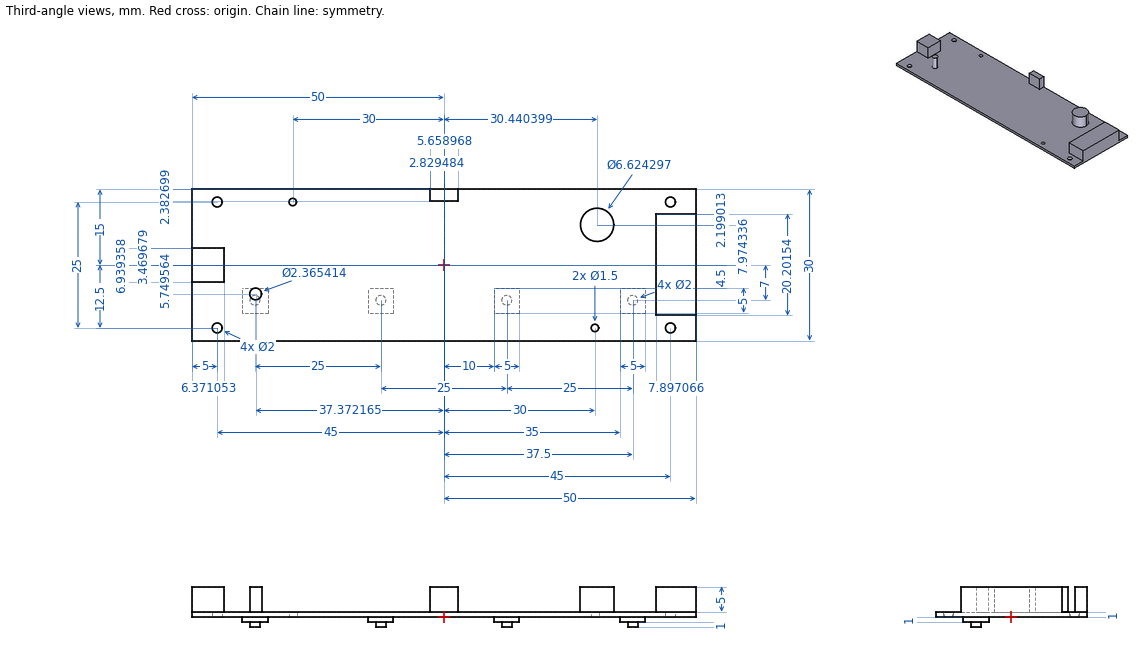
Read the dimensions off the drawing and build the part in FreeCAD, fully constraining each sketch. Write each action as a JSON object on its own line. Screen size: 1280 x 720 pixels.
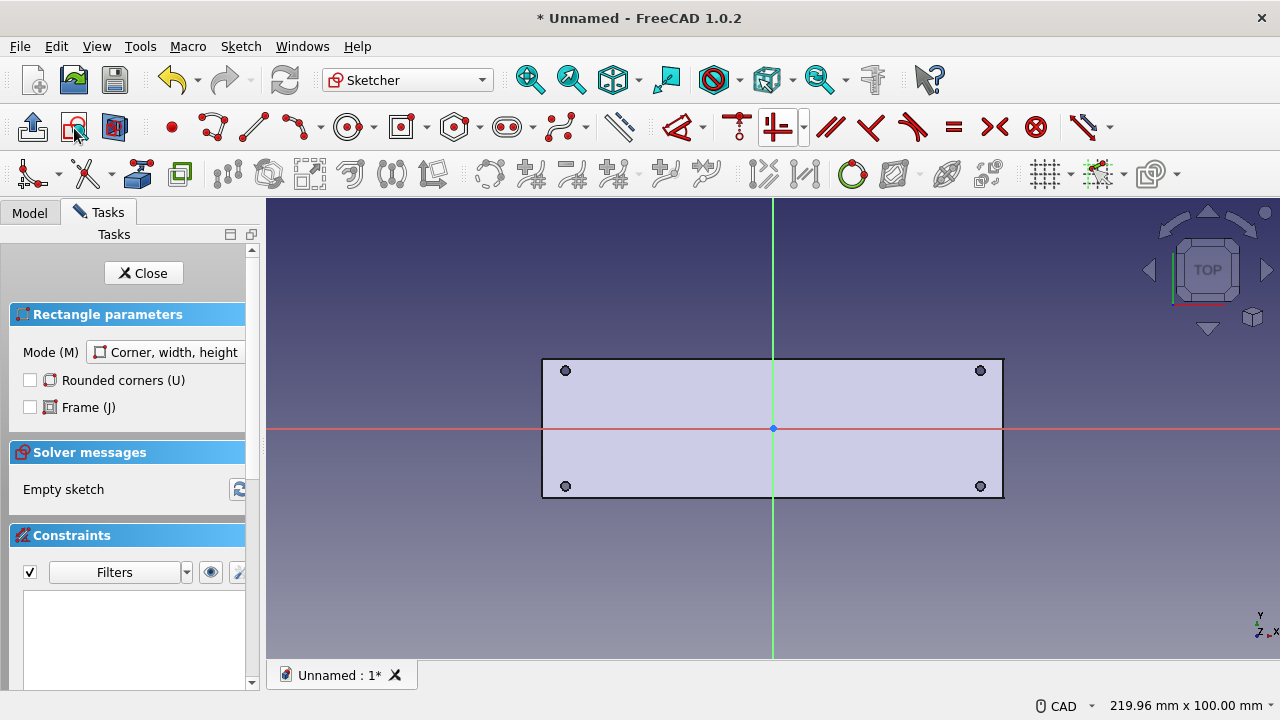
{"action": "left_click", "coordinate": [967, 382]}
{"action": "left_click", "coordinate": [1003, 475]}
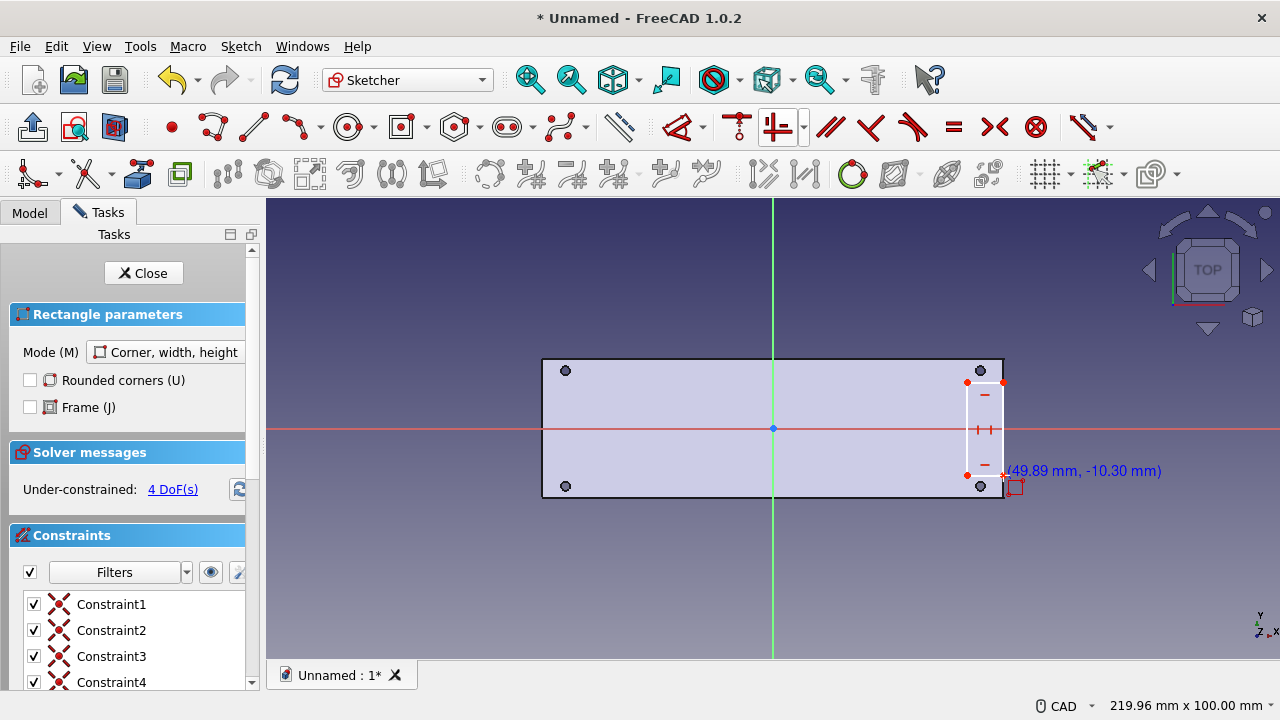
{"action": "scroll", "coordinate": [760, 359], "scroll_direction": "up", "scroll_amount": 2}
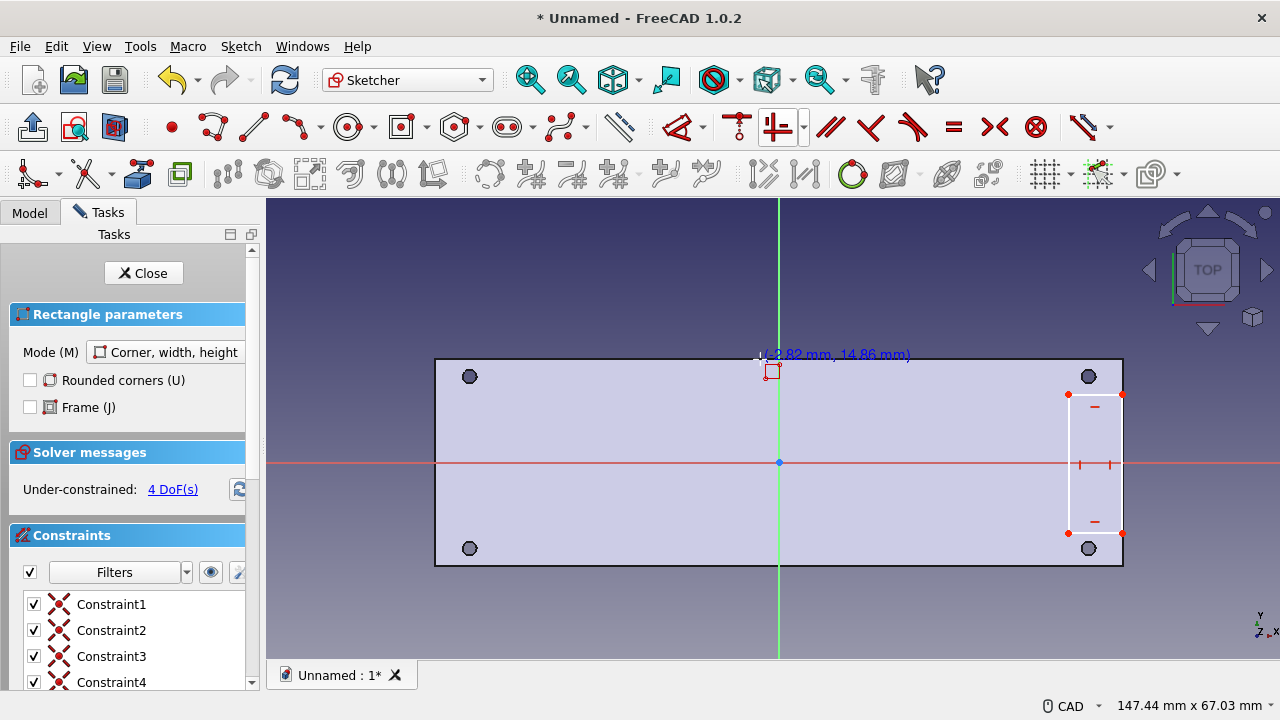
{"action": "left_click", "coordinate": [760, 359]}
{"action": "left_click", "coordinate": [799, 376]}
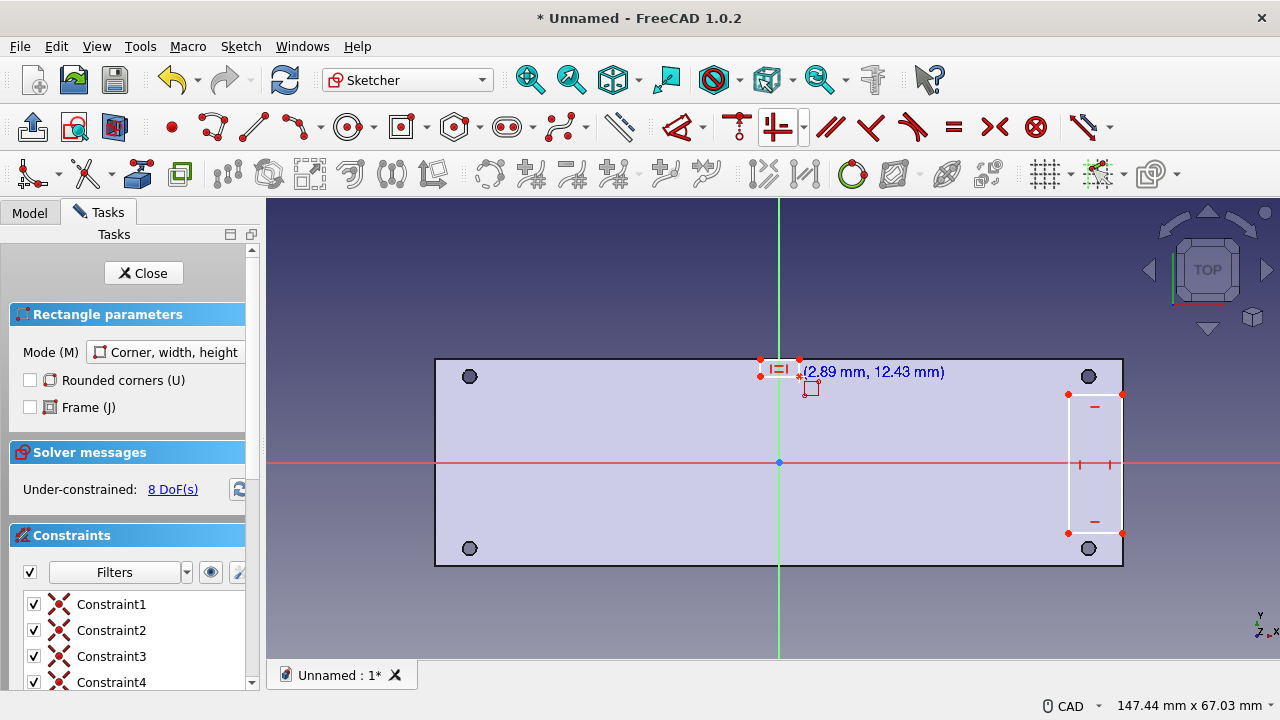
{"action": "left_click", "coordinate": [435, 439]}
{"action": "left_click", "coordinate": [479, 486]}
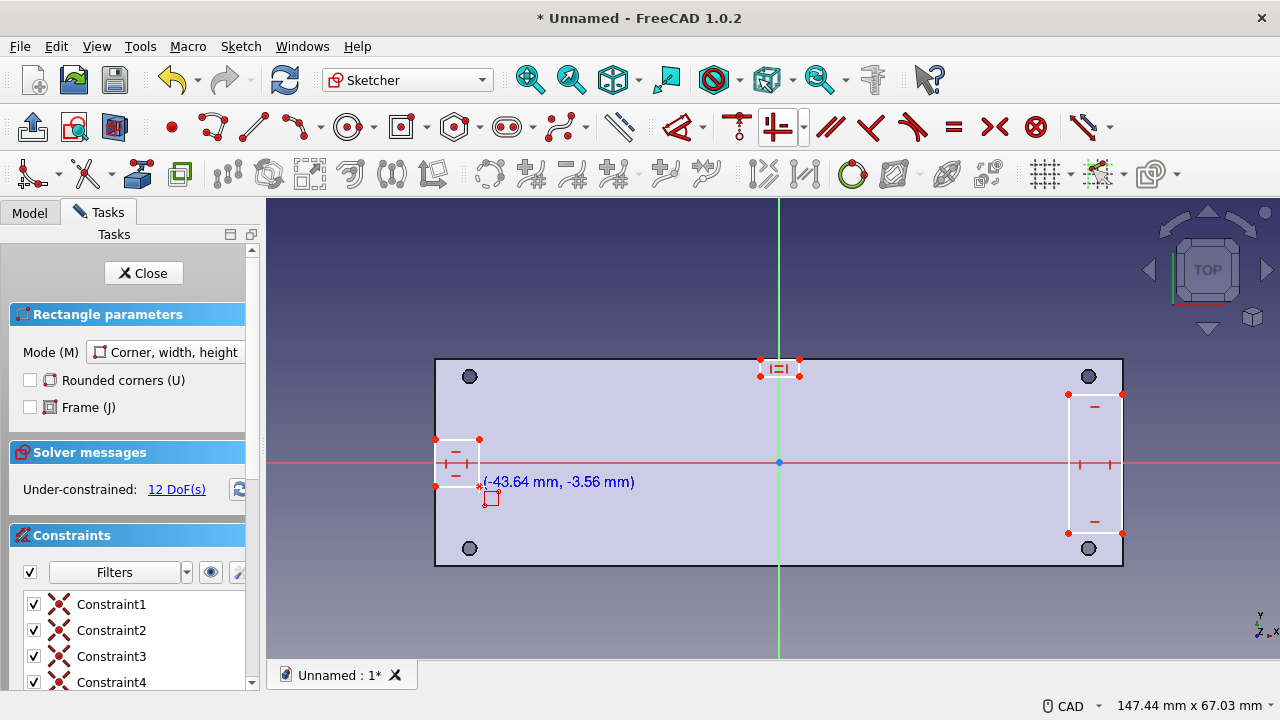
{"action": "left_click", "coordinate": [348, 128]}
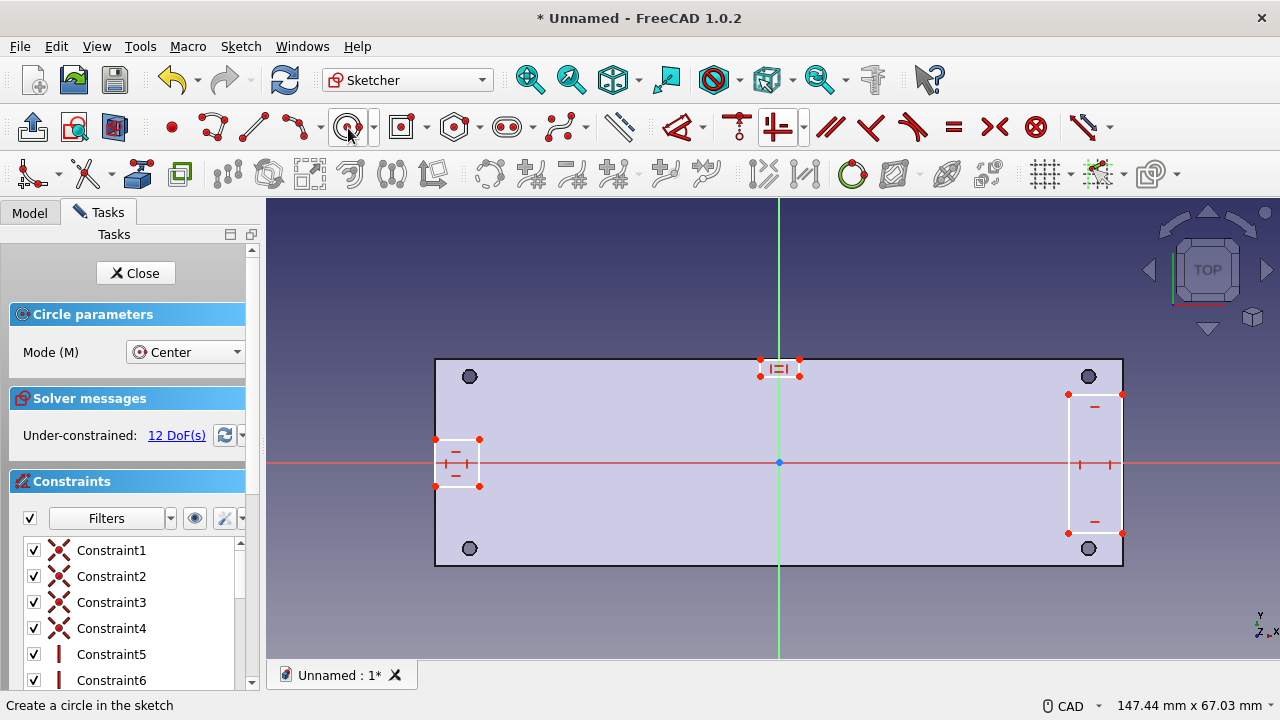
{"action": "left_click", "coordinate": [989, 408]}
{"action": "left_click", "coordinate": [1005, 392]}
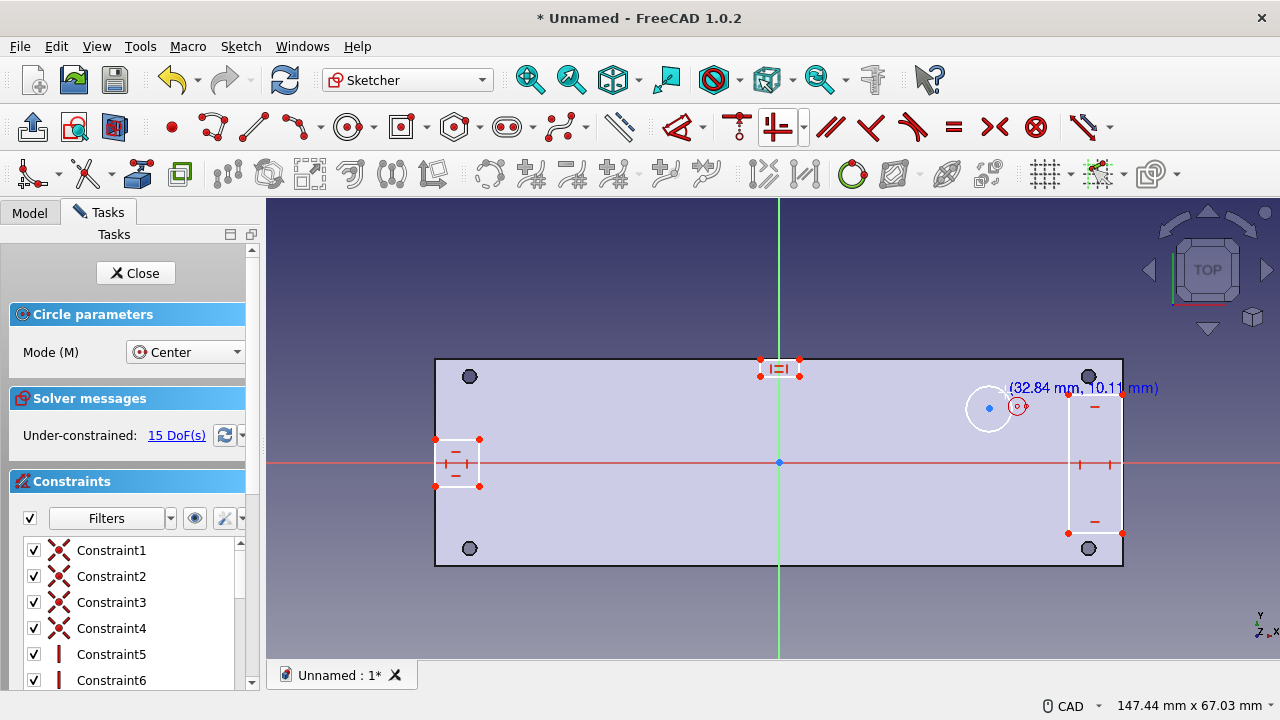
{"action": "scroll", "coordinate": [522, 502], "scroll_direction": "up", "scroll_amount": 6}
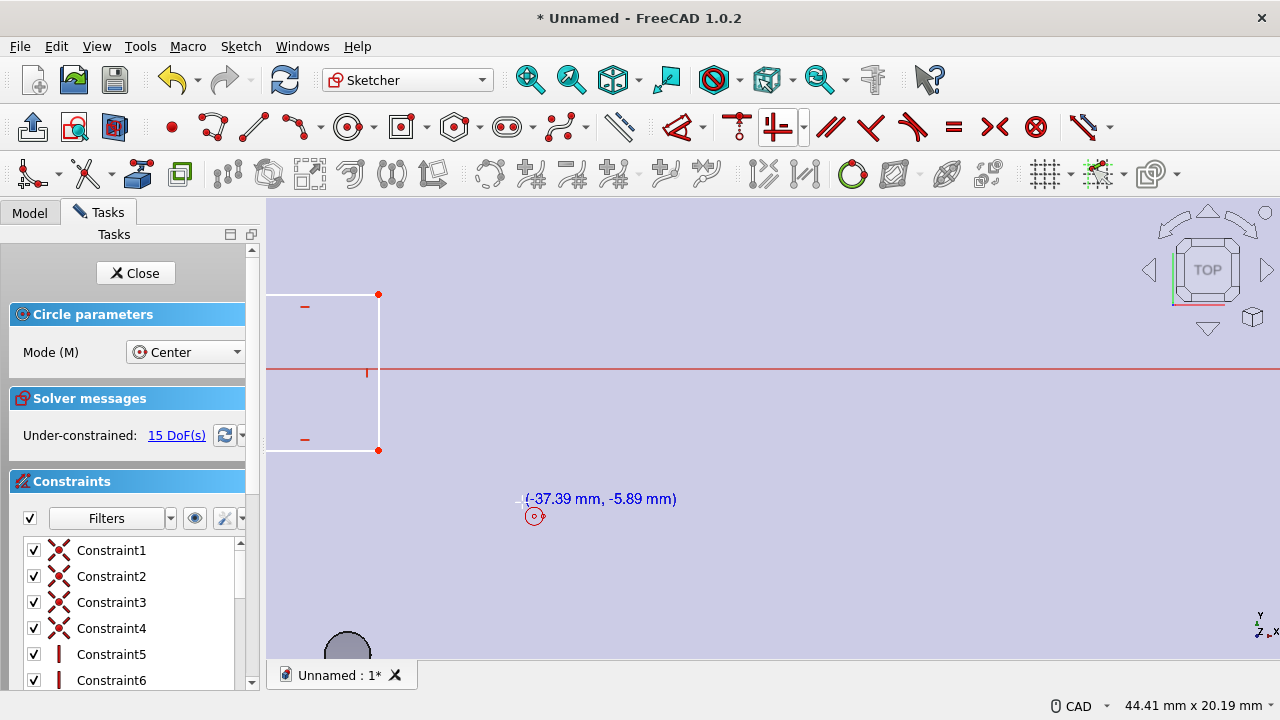
{"action": "scroll", "coordinate": [485, 466], "scroll_direction": "down", "scroll_amount": 7}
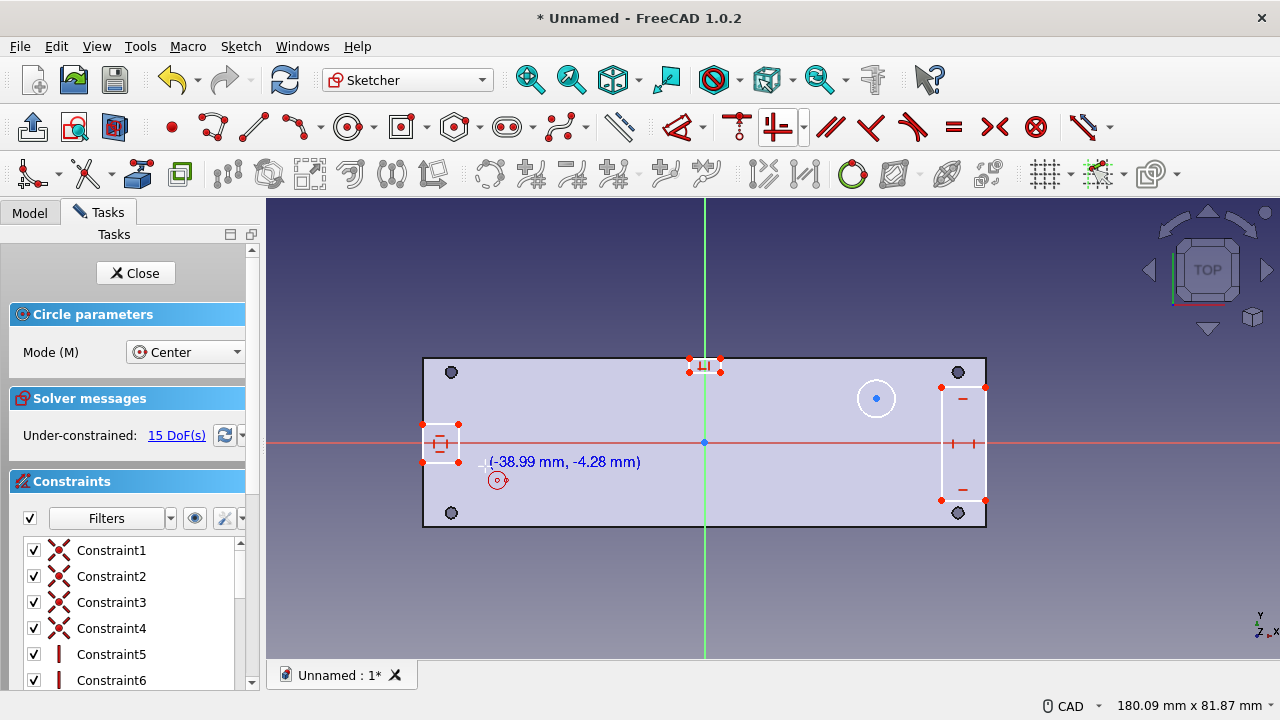
{"action": "left_click", "coordinate": [494, 475]}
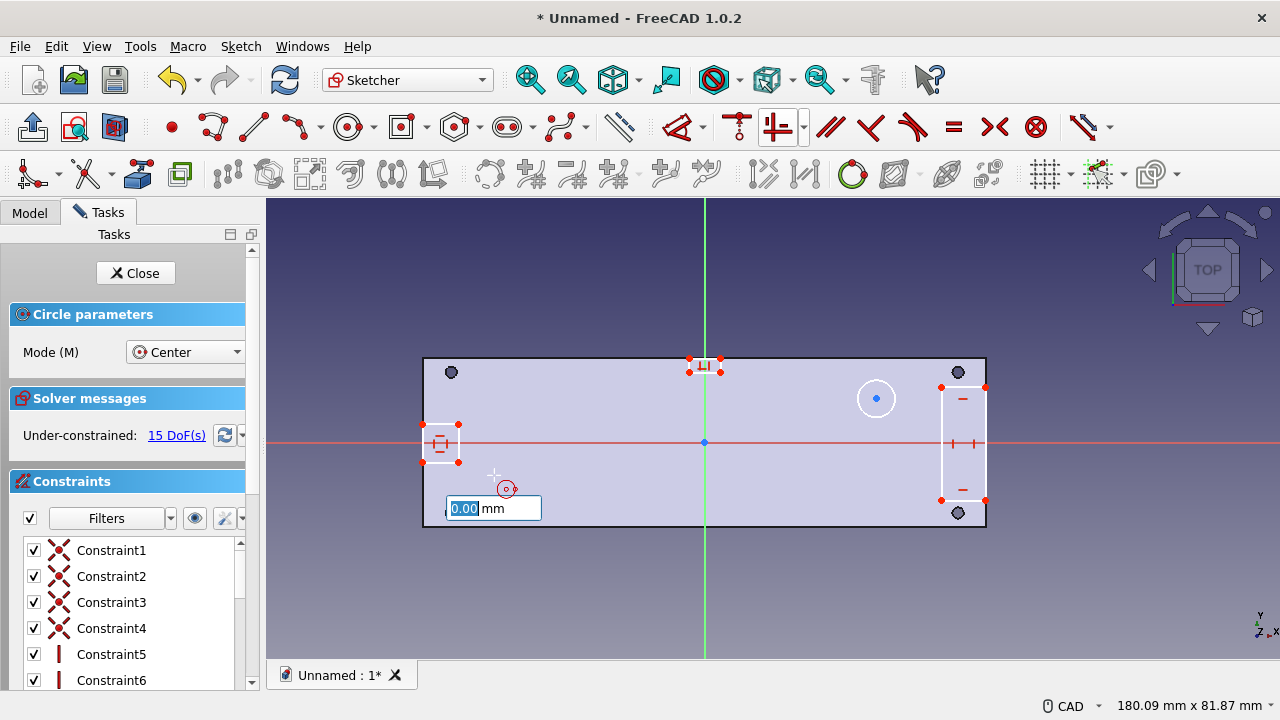
{"action": "scroll", "coordinate": [499, 470], "scroll_direction": "up", "scroll_amount": 5}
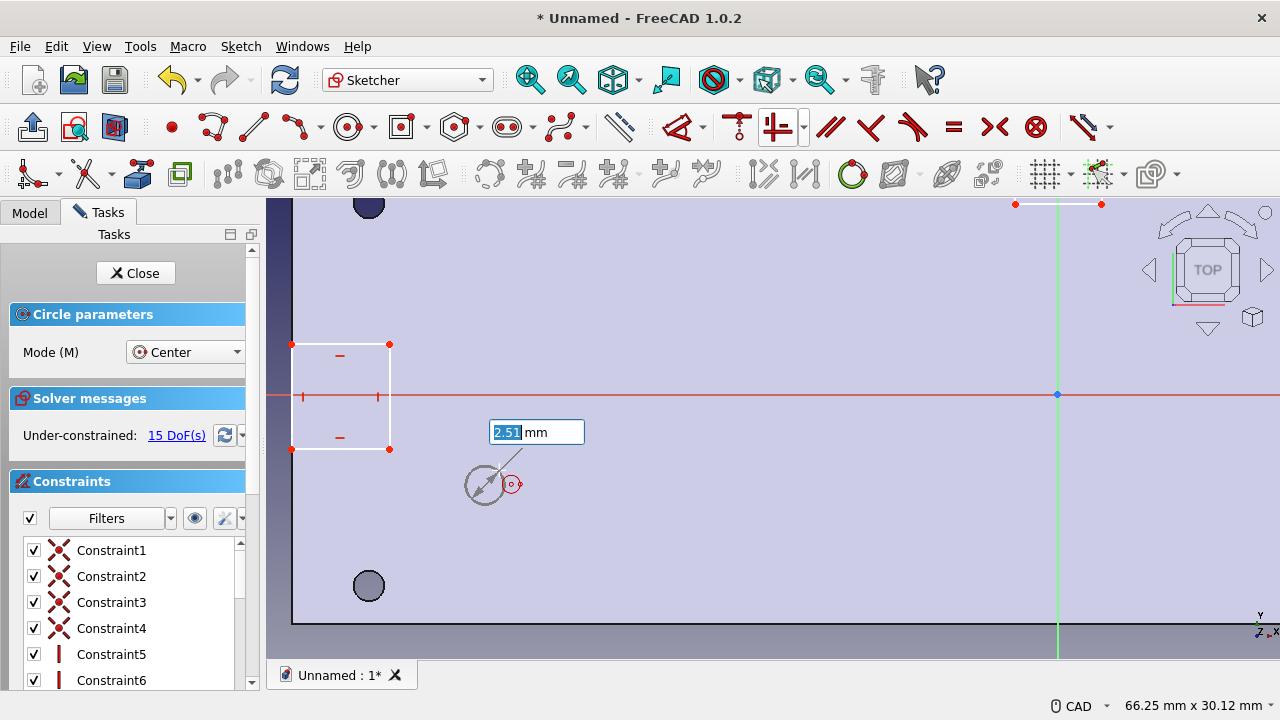
{"action": "left_click", "coordinate": [498, 470]}
{"action": "key", "text": "Escape"}